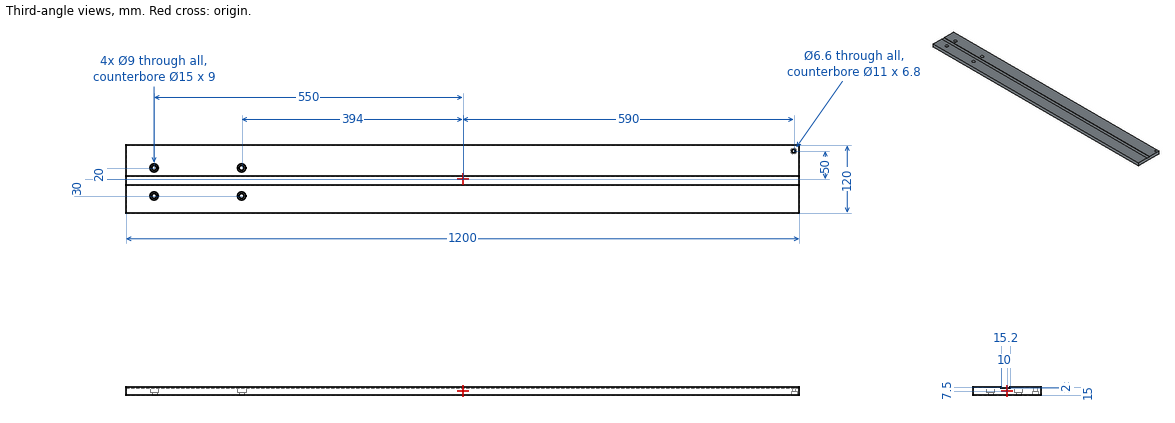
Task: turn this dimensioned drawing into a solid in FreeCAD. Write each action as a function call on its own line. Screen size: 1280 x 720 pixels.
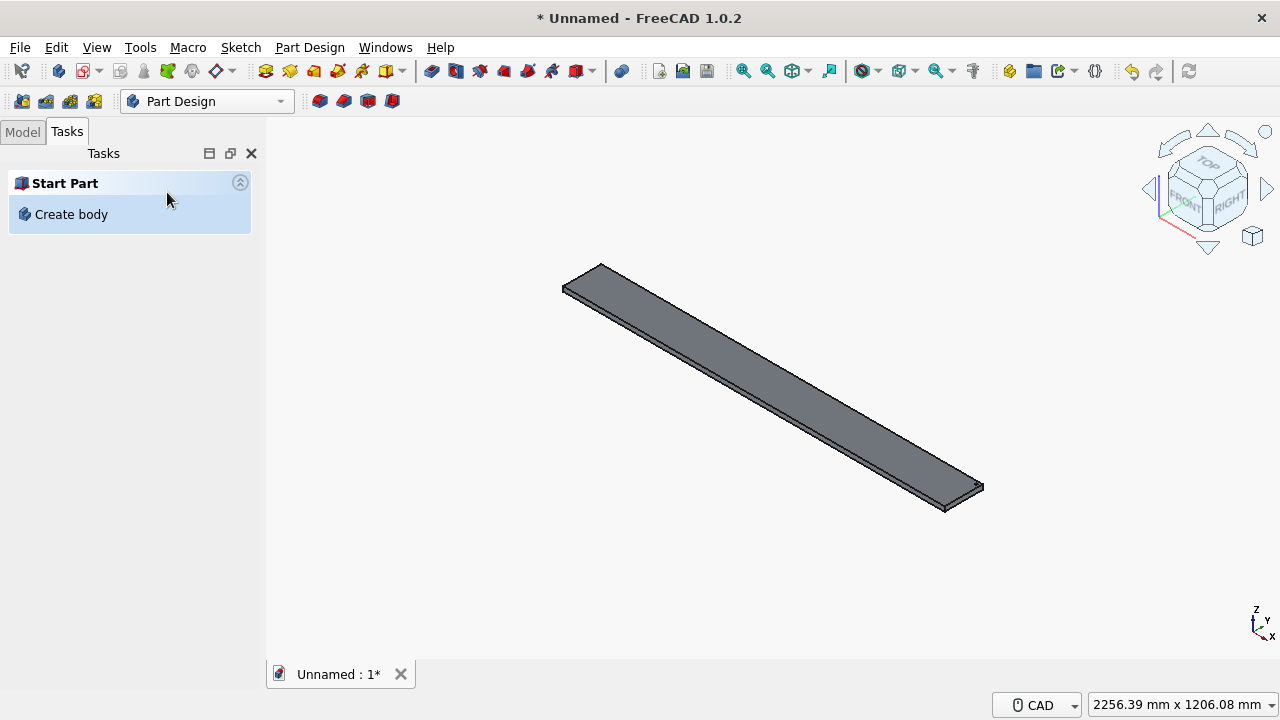
click(936, 479)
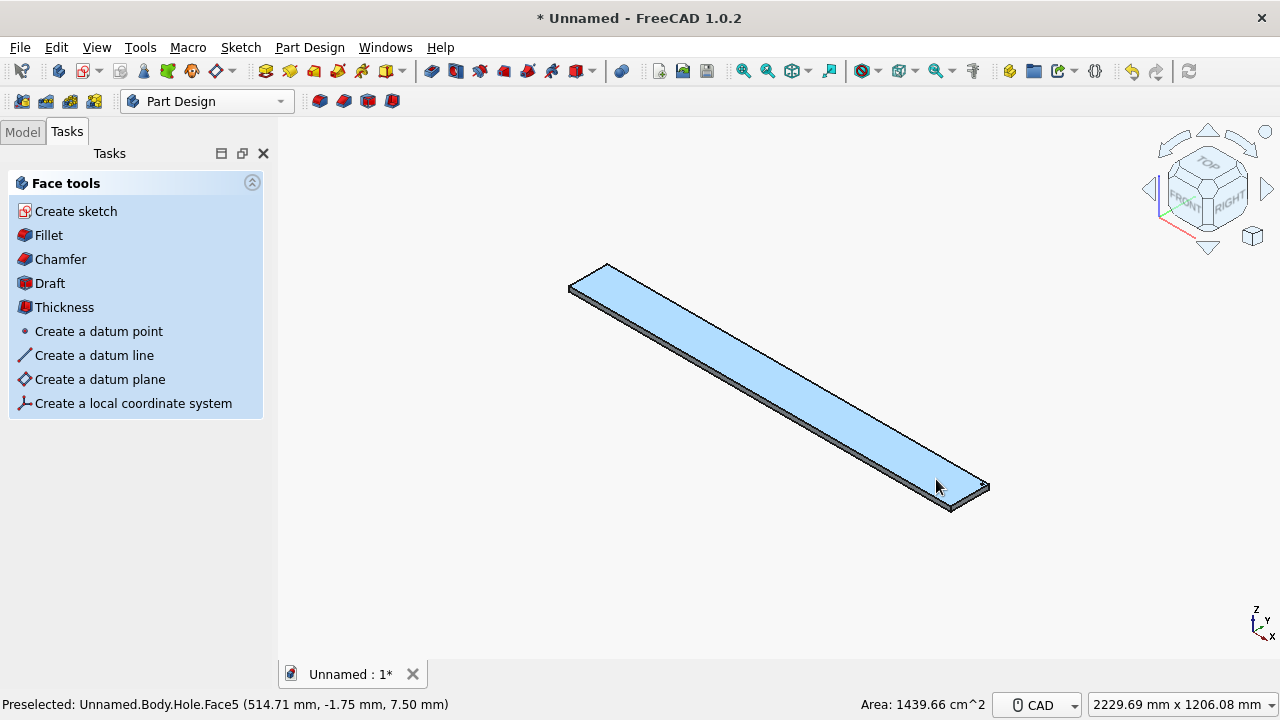
click(84, 72)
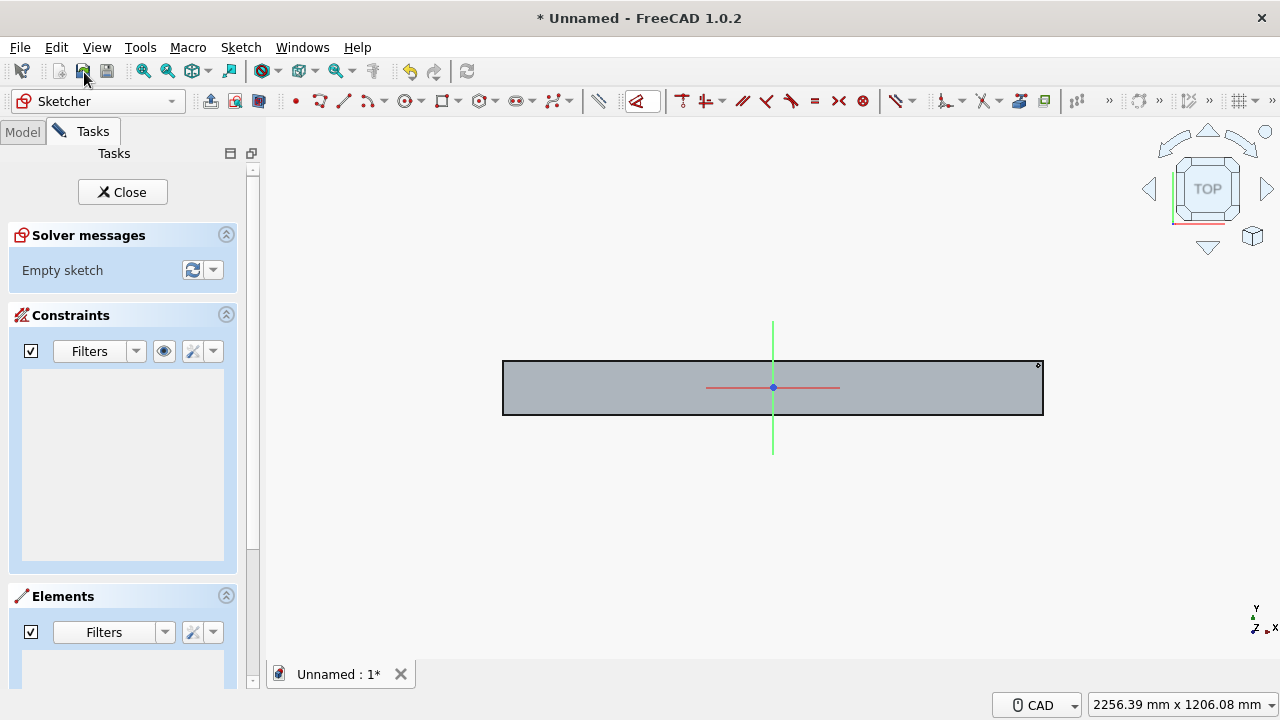
scroll(538, 391, up, 10)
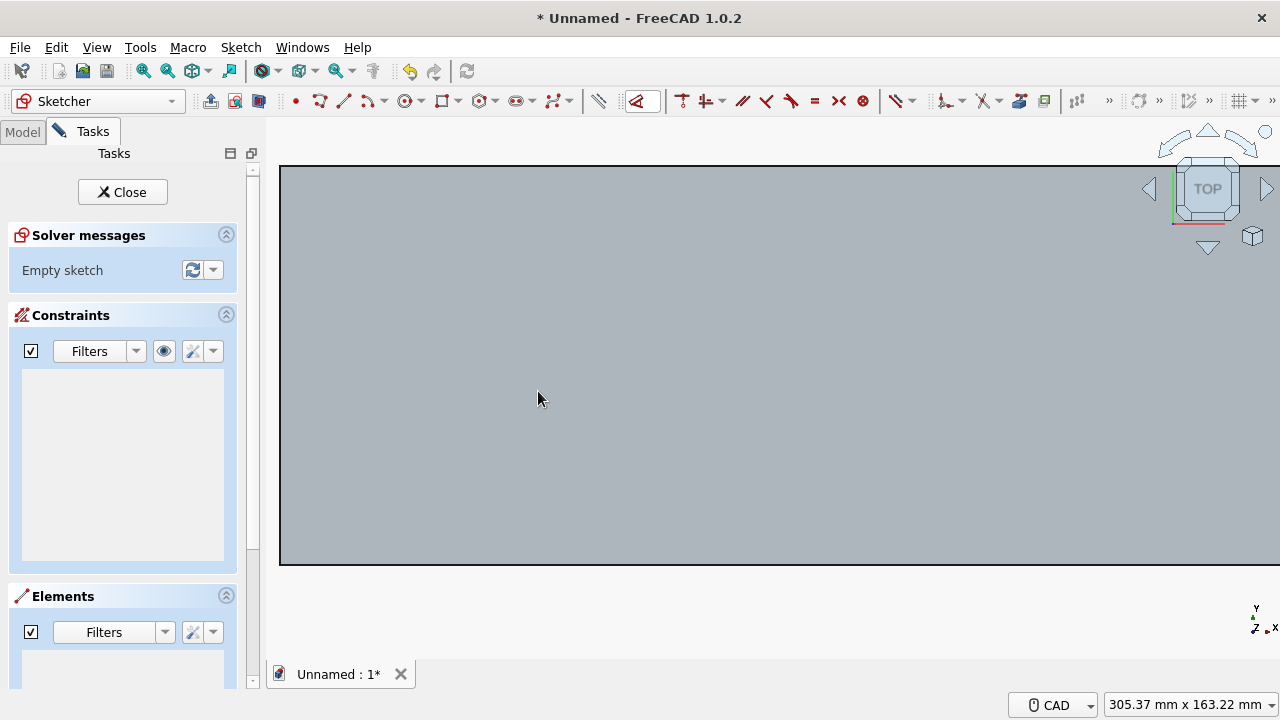
click(406, 102)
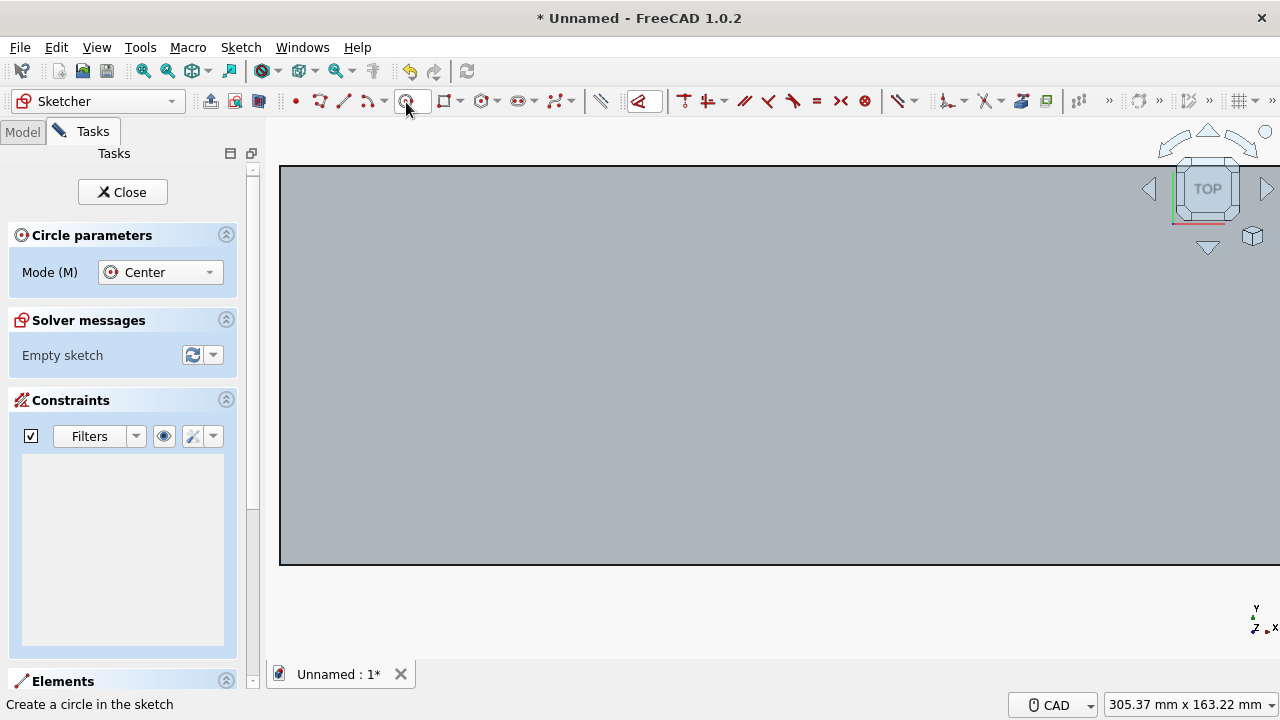
scroll(446, 299, up, 3)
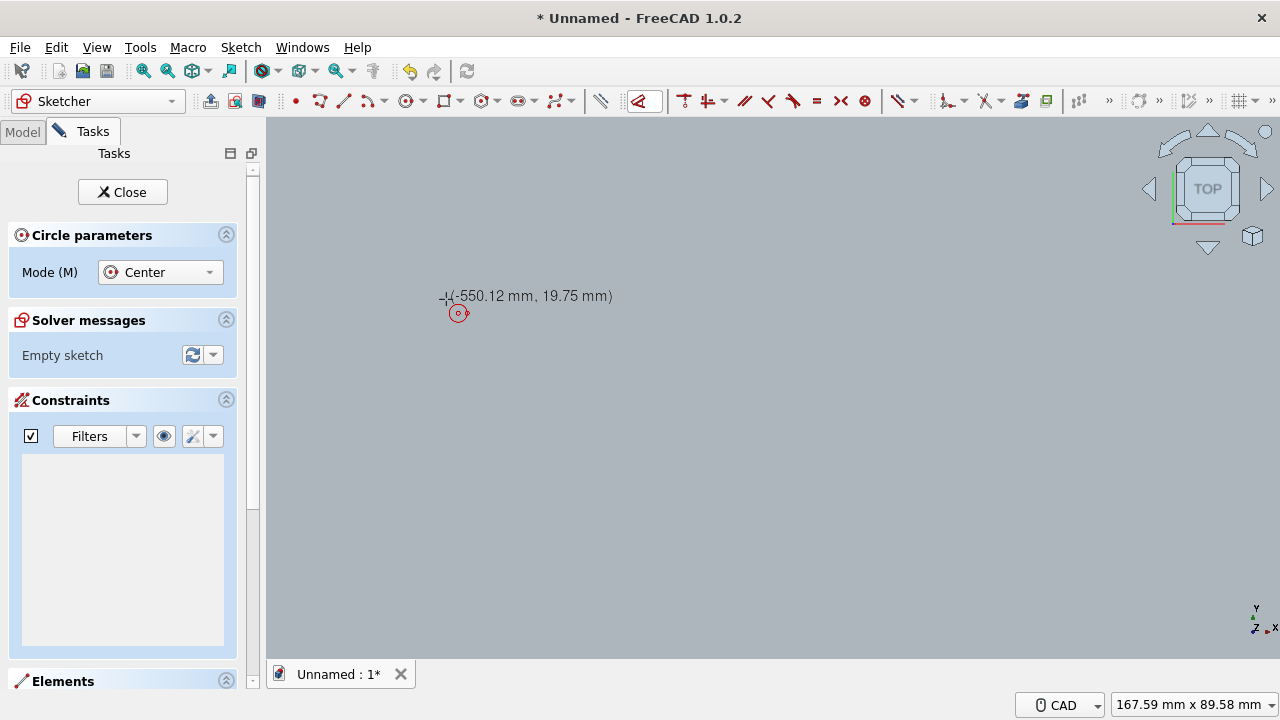
click(447, 299)
move(466, 280)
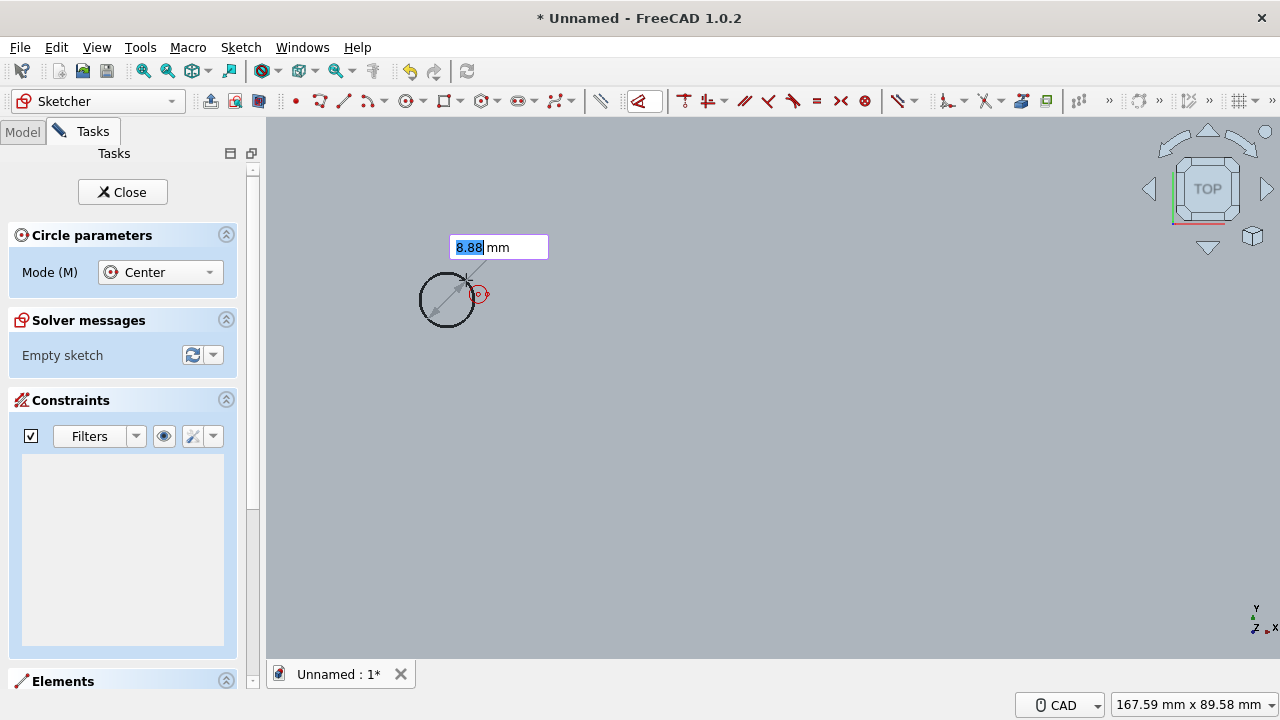
text(9)
key(Return)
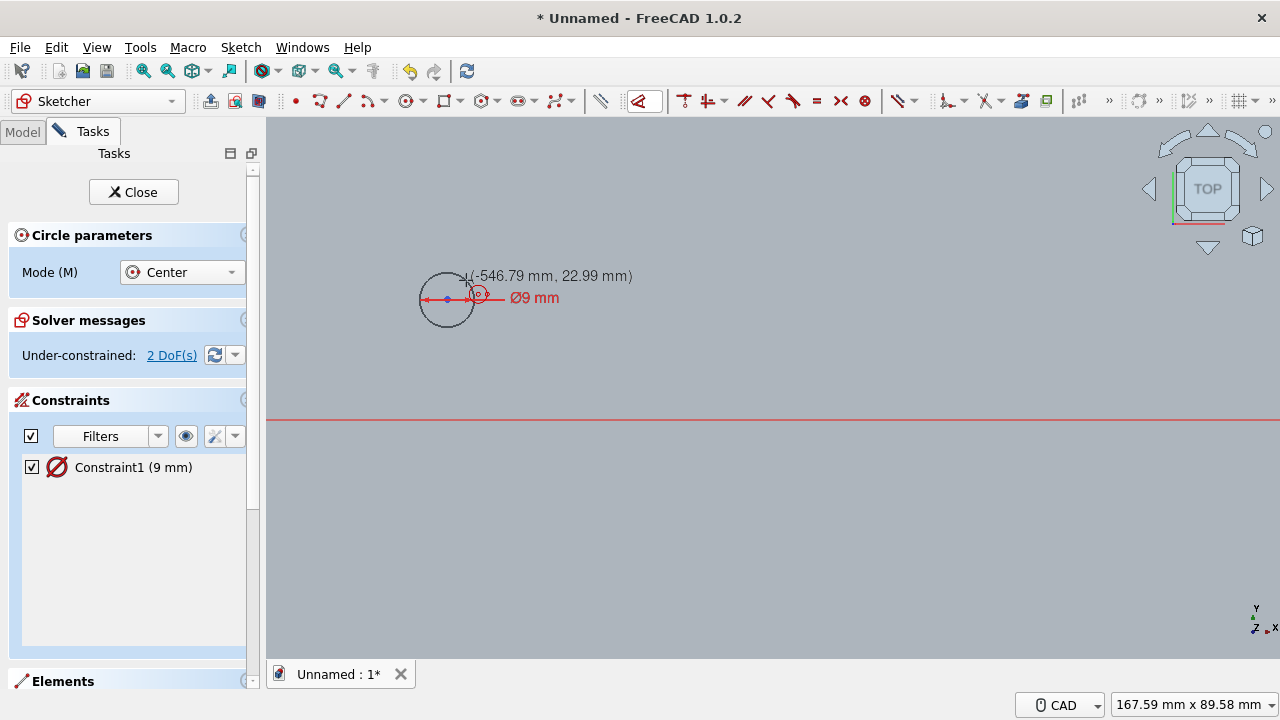
scroll(444, 312, down, 3)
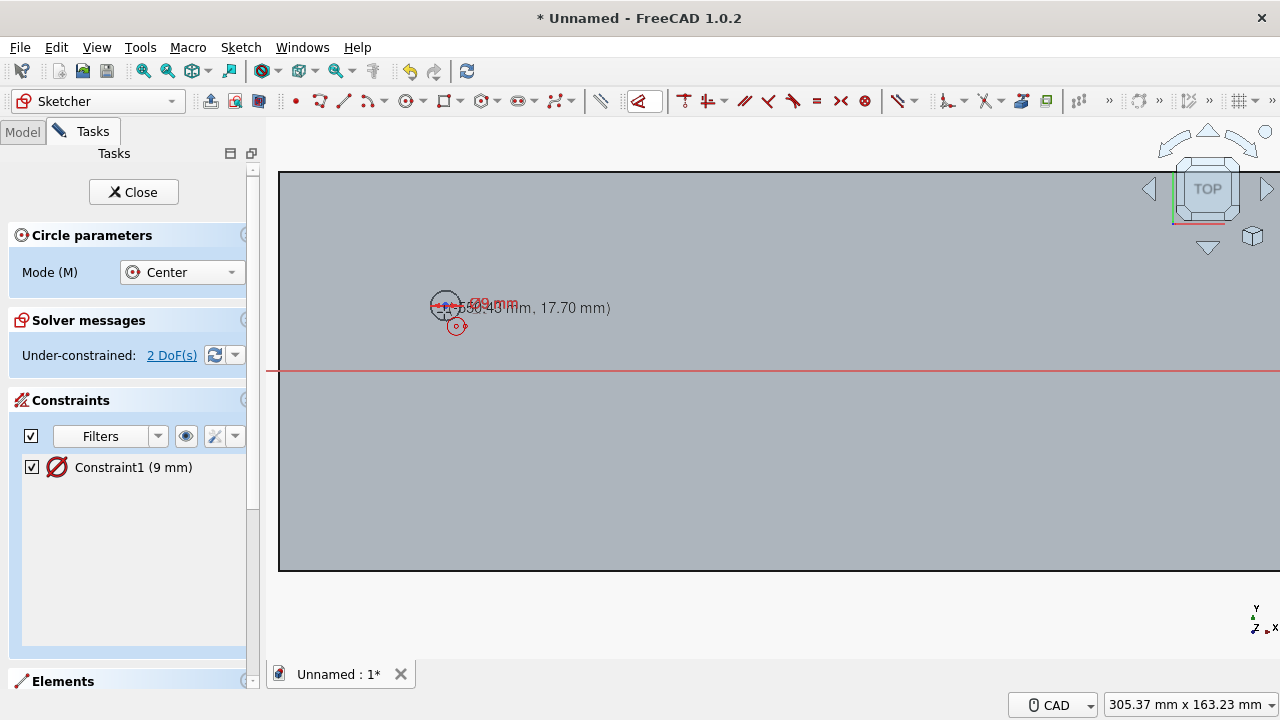
scroll(964, 305, up, 3)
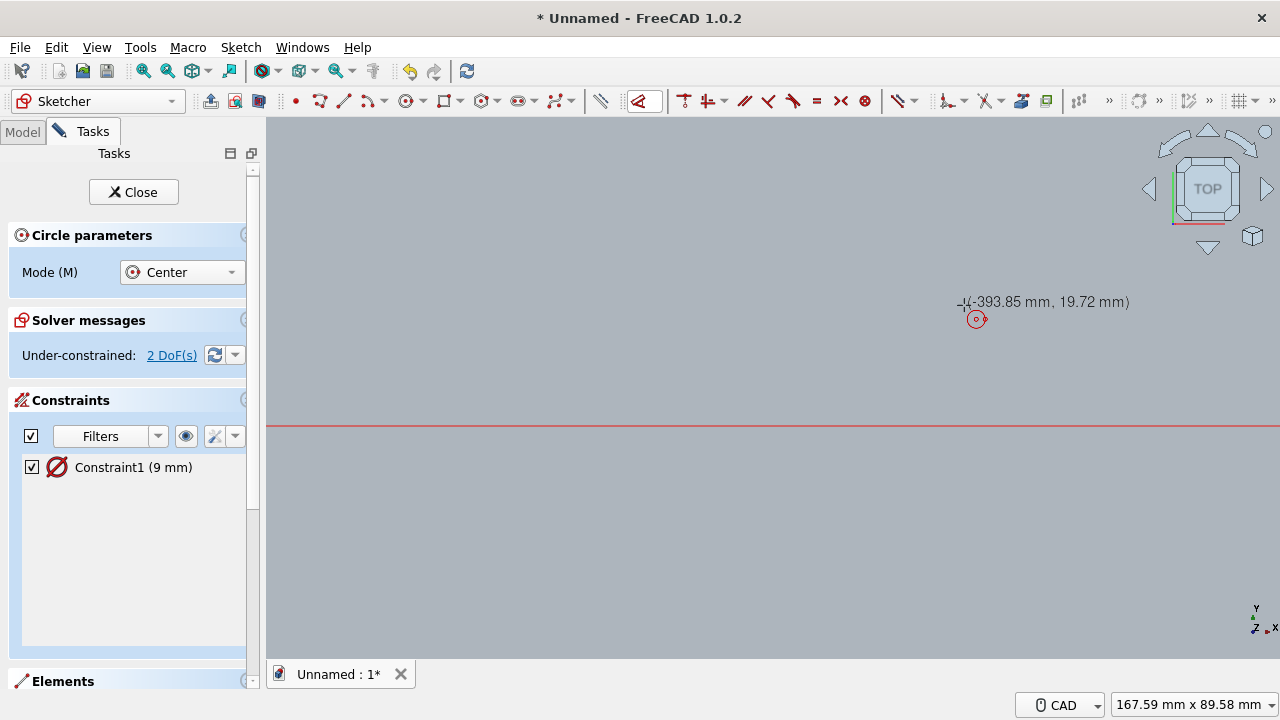
click(963, 305)
move(982, 286)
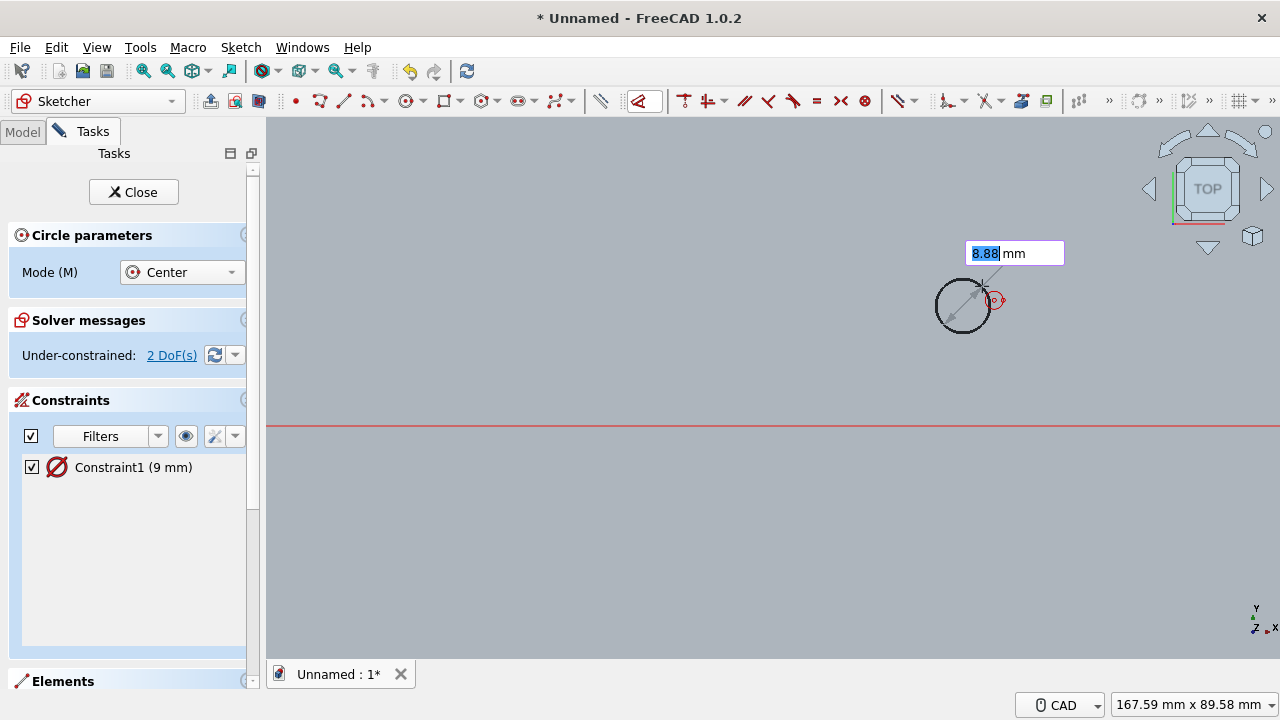
text(9)
key(Return)